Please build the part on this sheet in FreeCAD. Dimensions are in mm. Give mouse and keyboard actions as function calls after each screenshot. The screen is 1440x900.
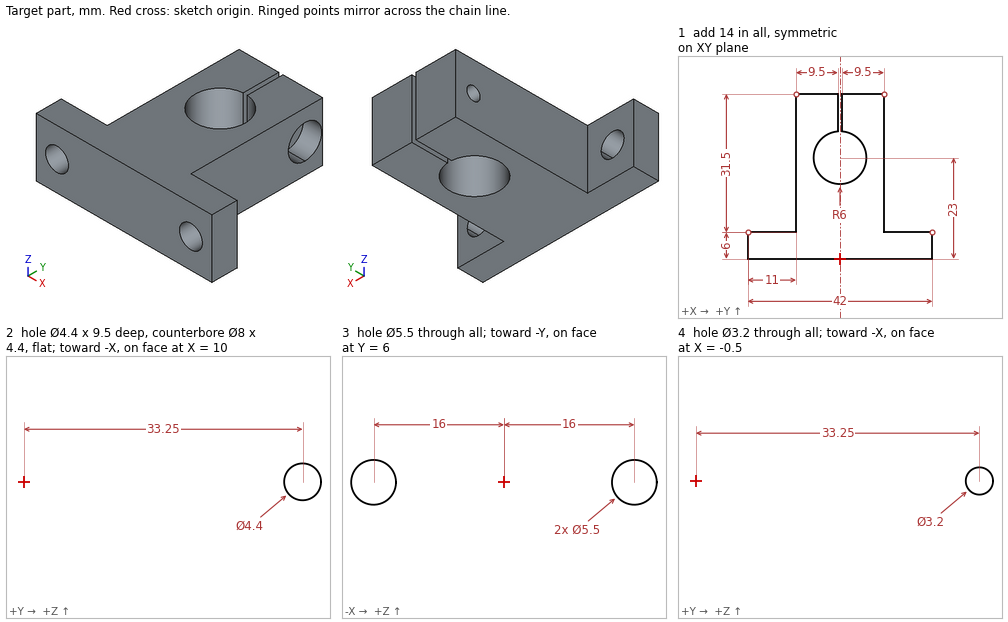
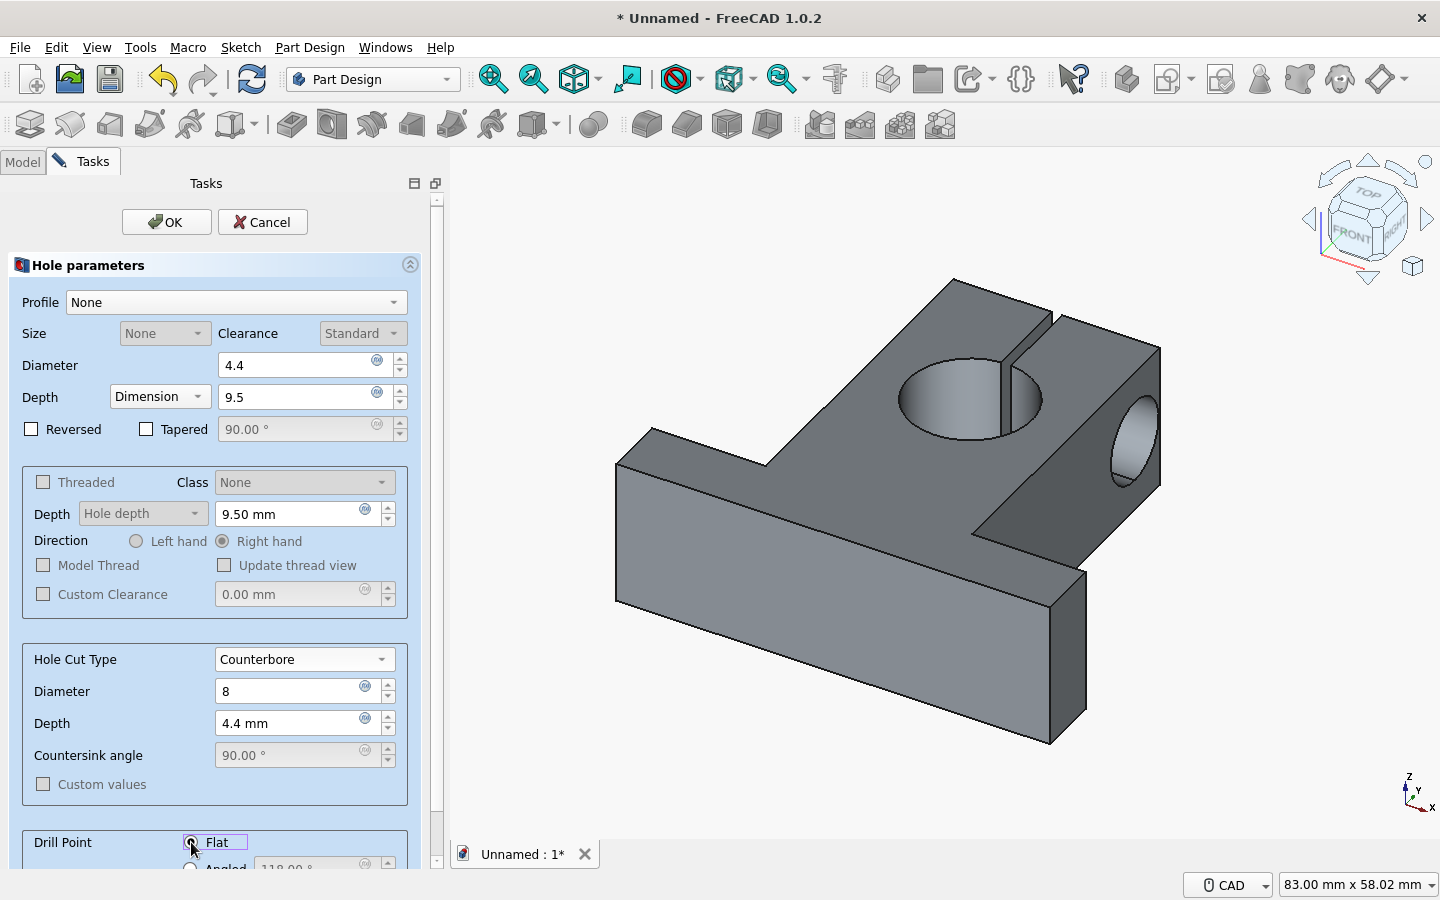
click(167, 222)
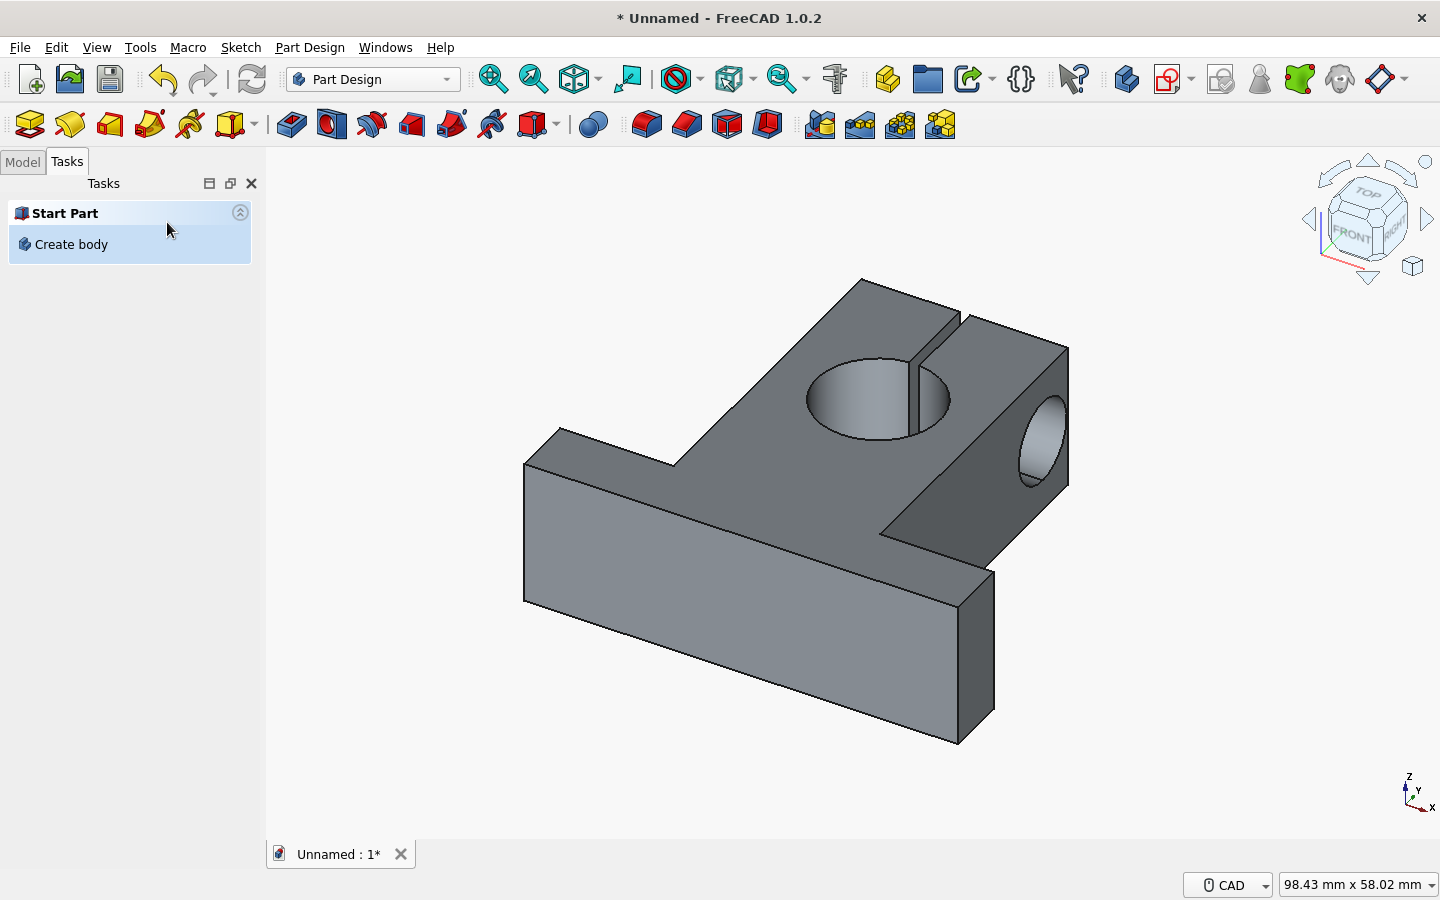
key(4)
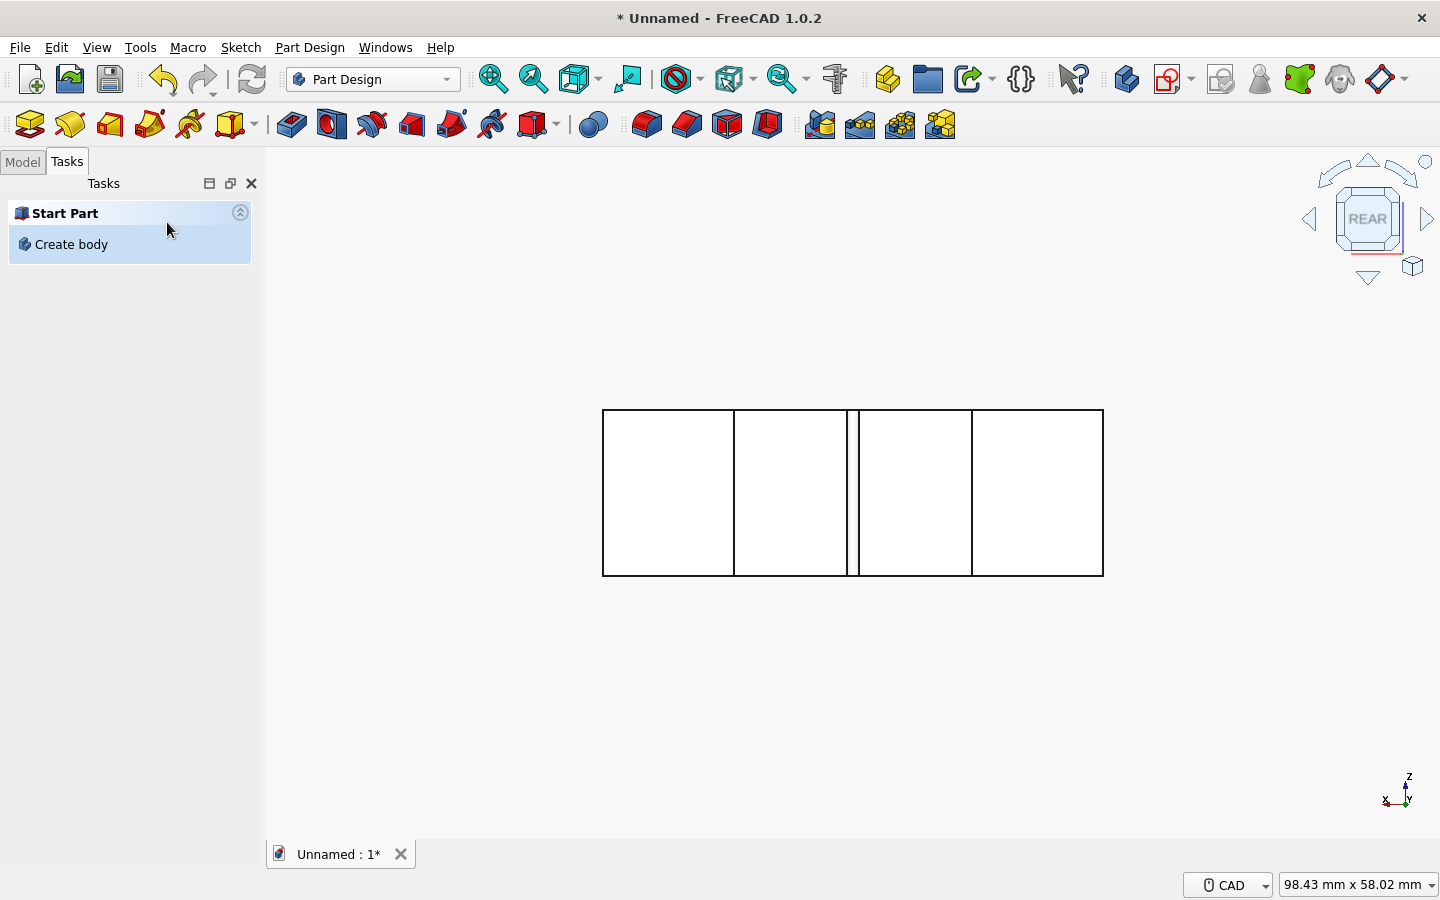
click(494, 80)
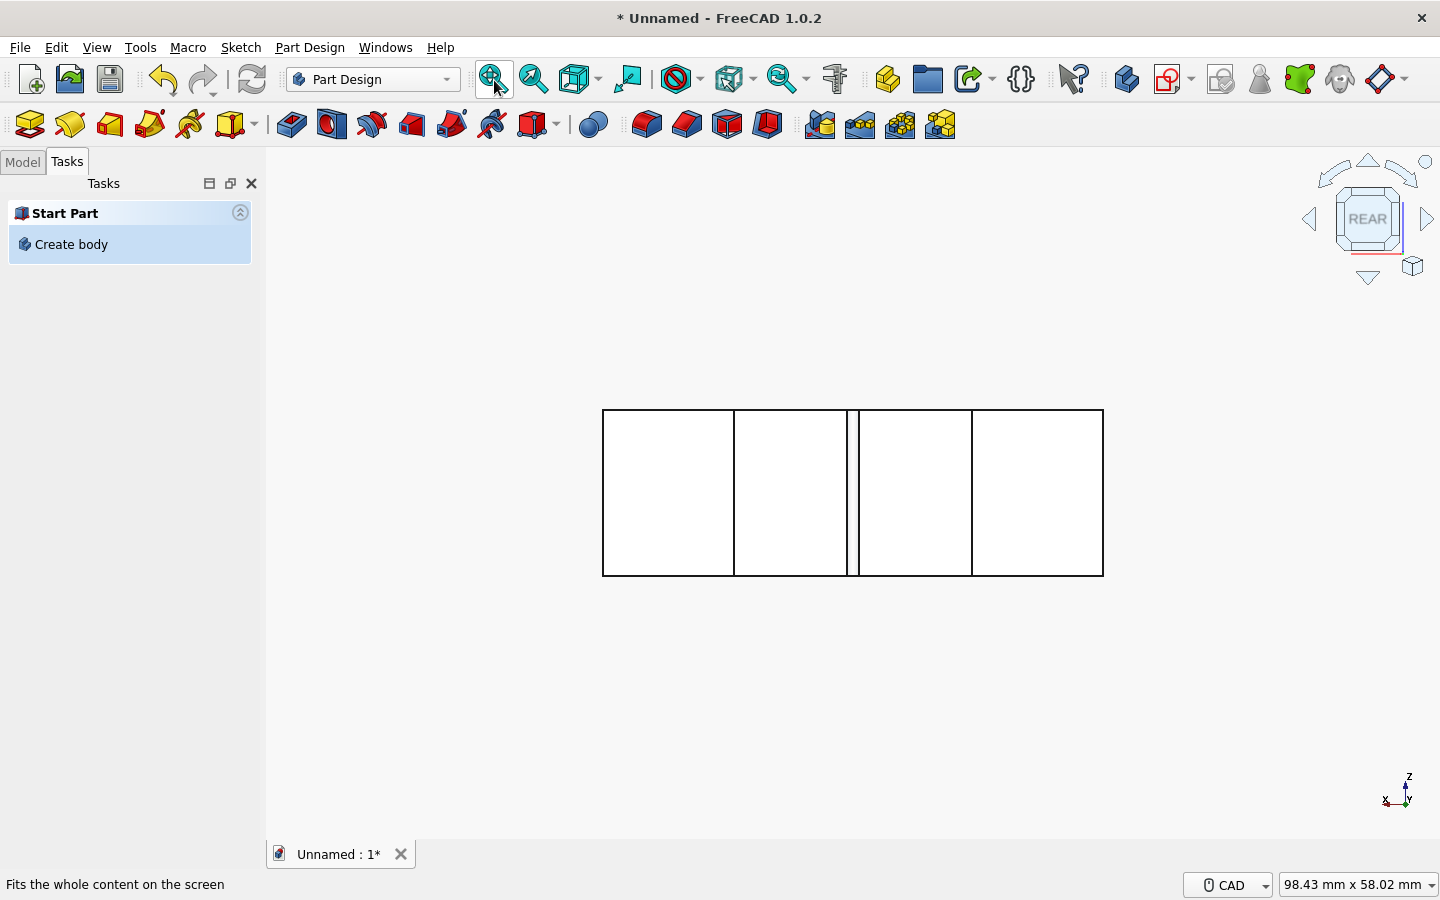
click(1038, 492)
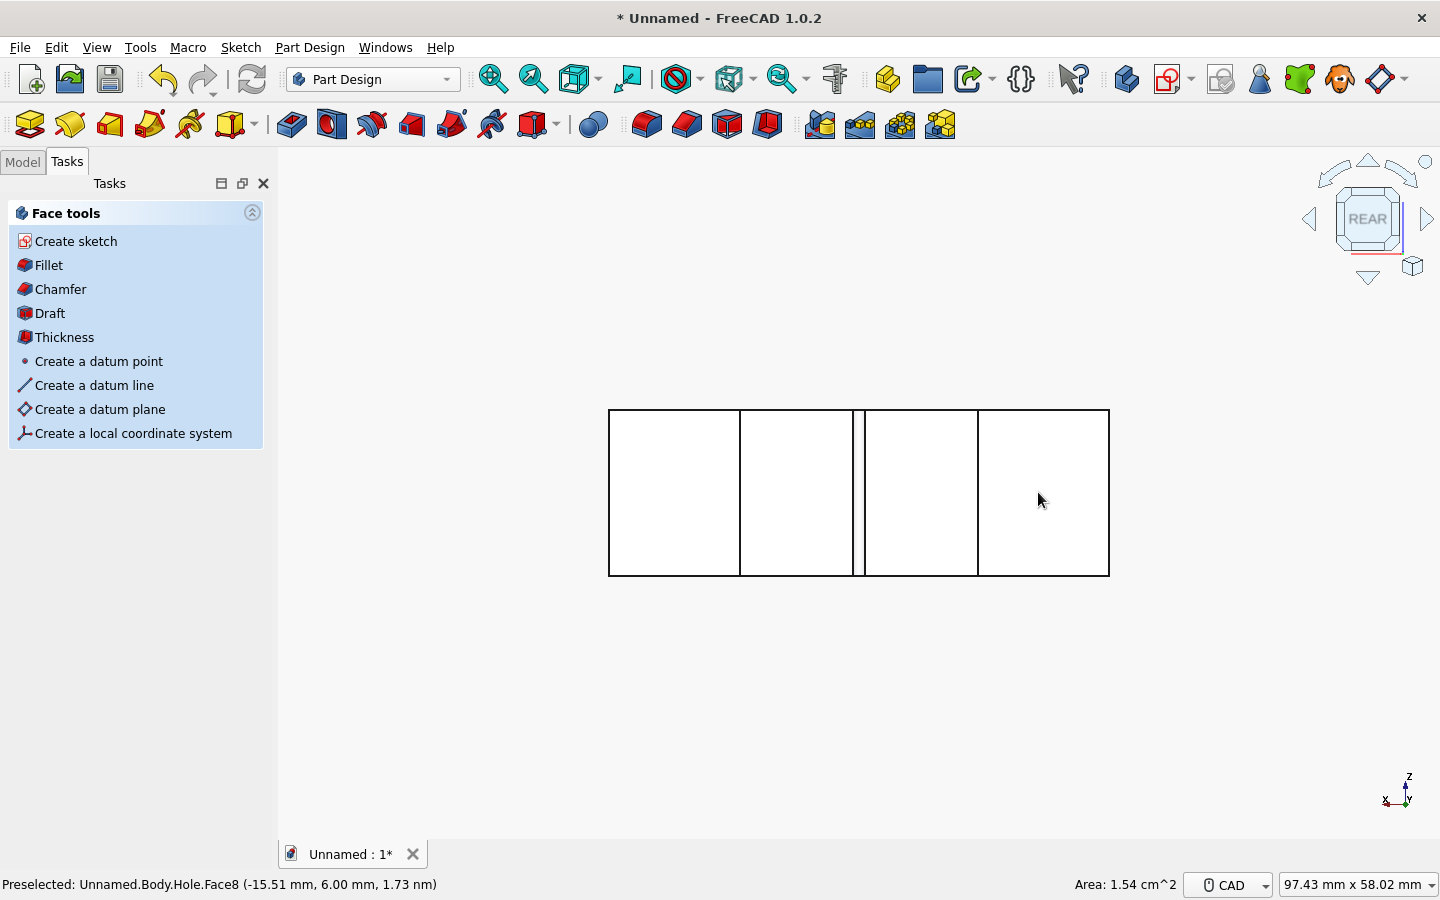
click(1168, 80)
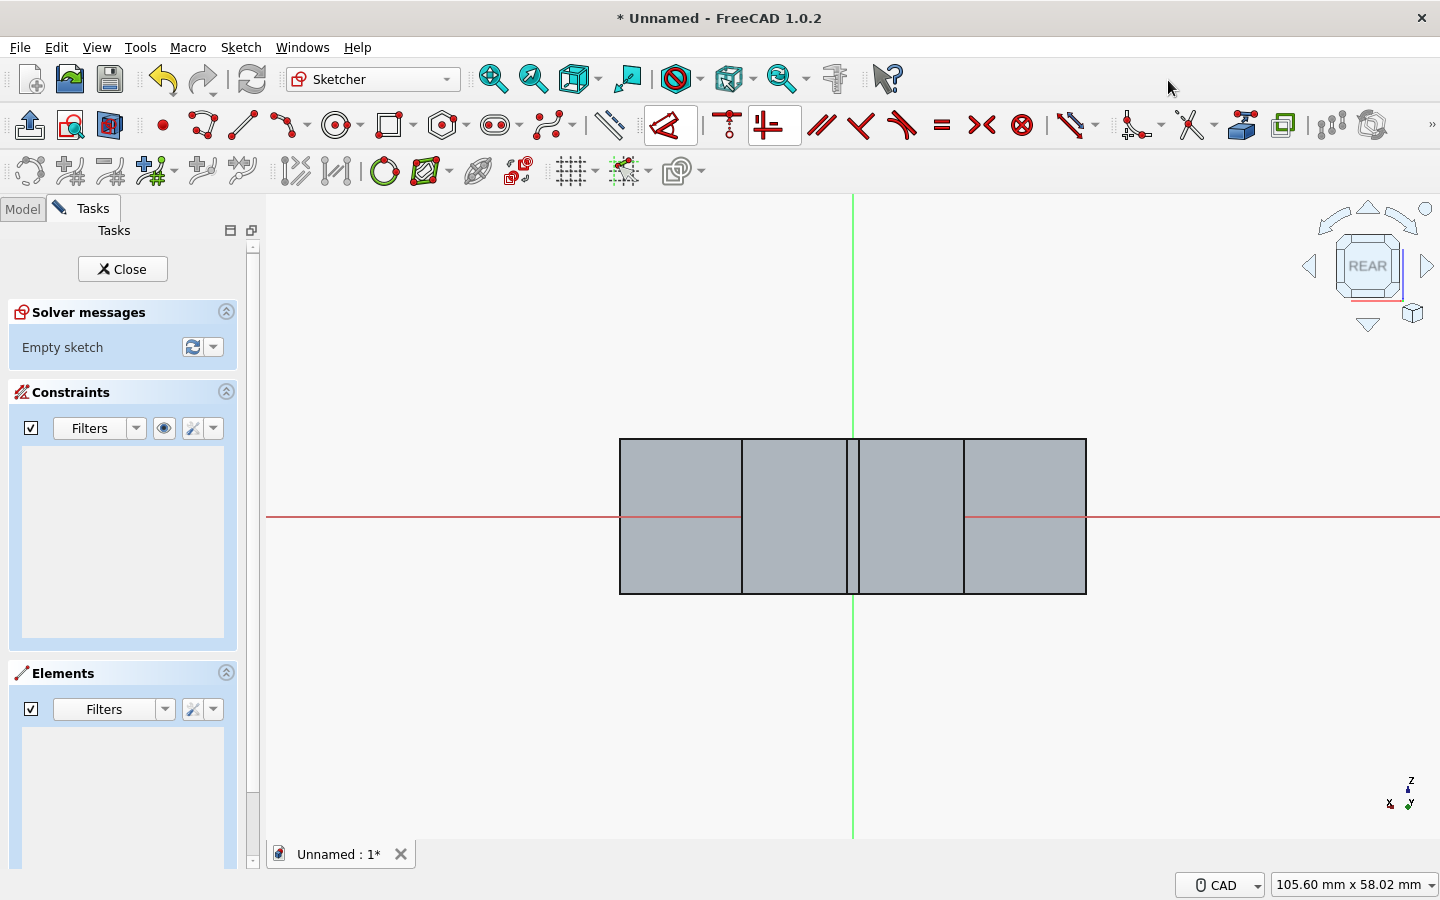
click(110, 126)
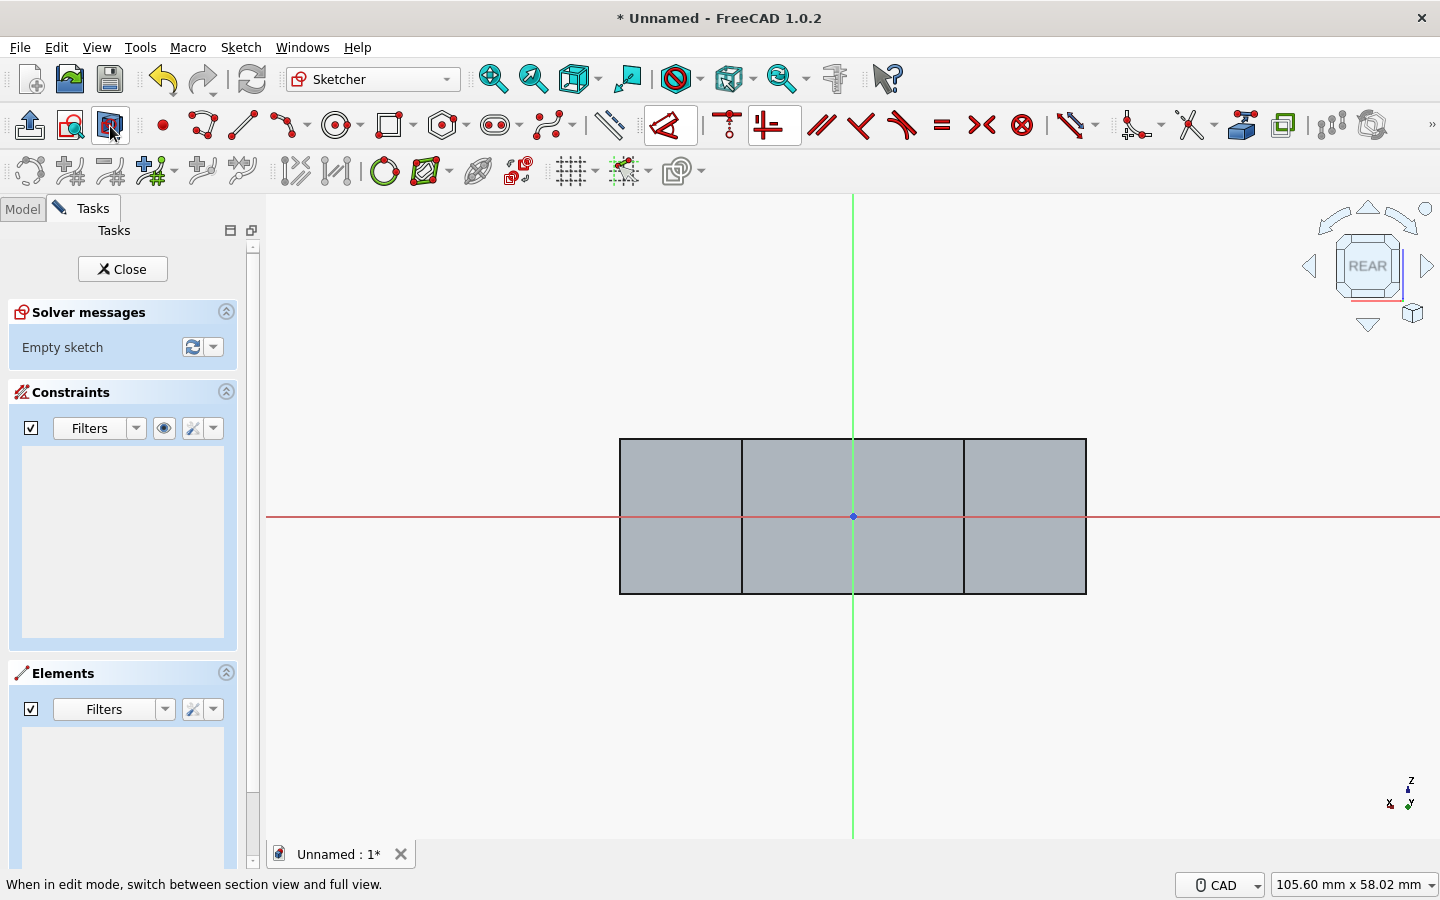
scroll(936, 517, up, 3)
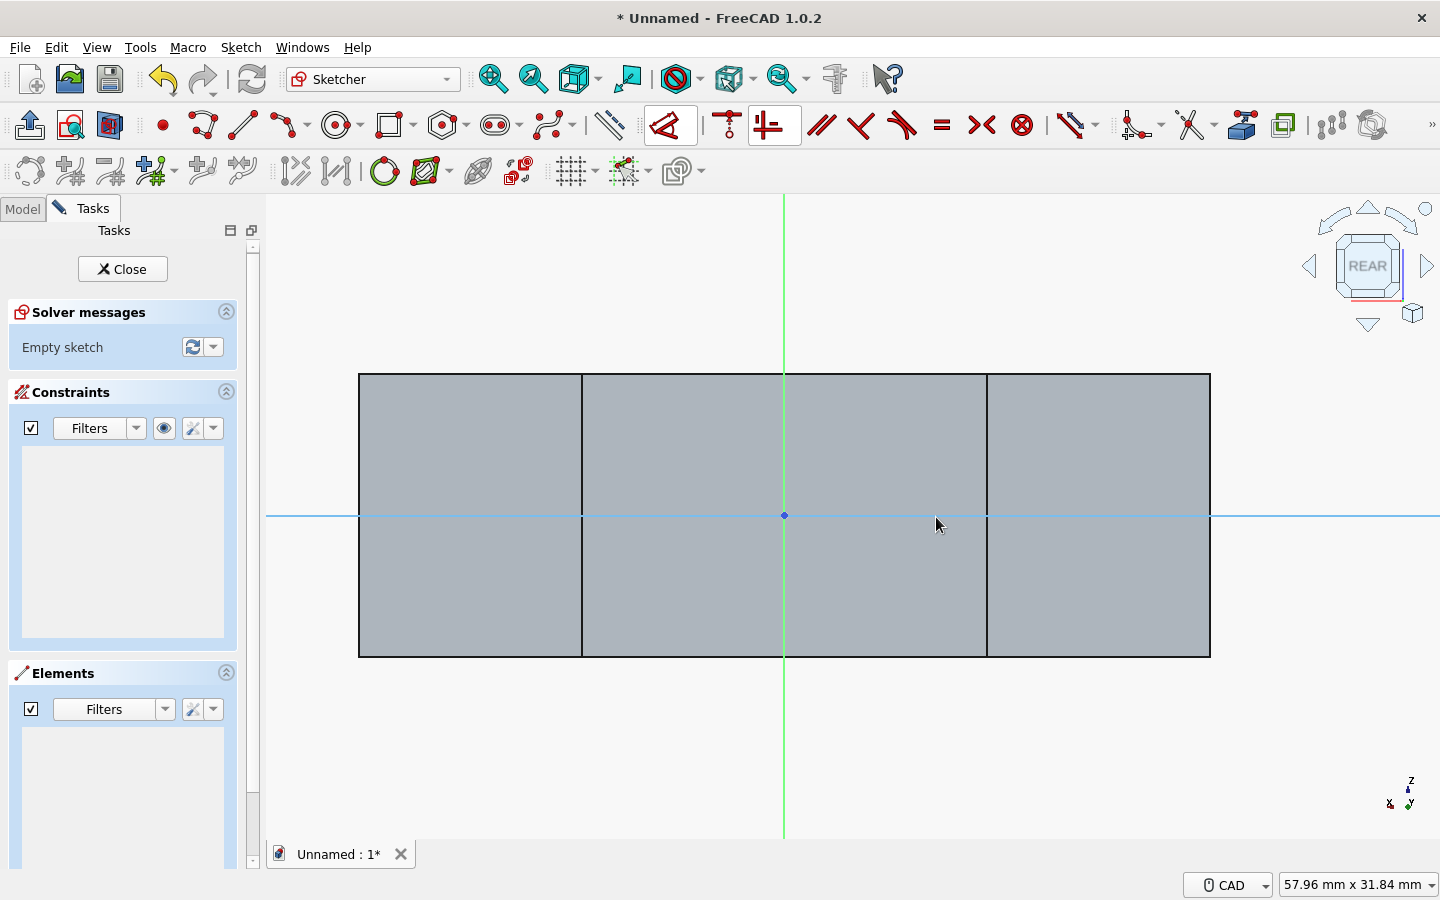
click(336, 126)